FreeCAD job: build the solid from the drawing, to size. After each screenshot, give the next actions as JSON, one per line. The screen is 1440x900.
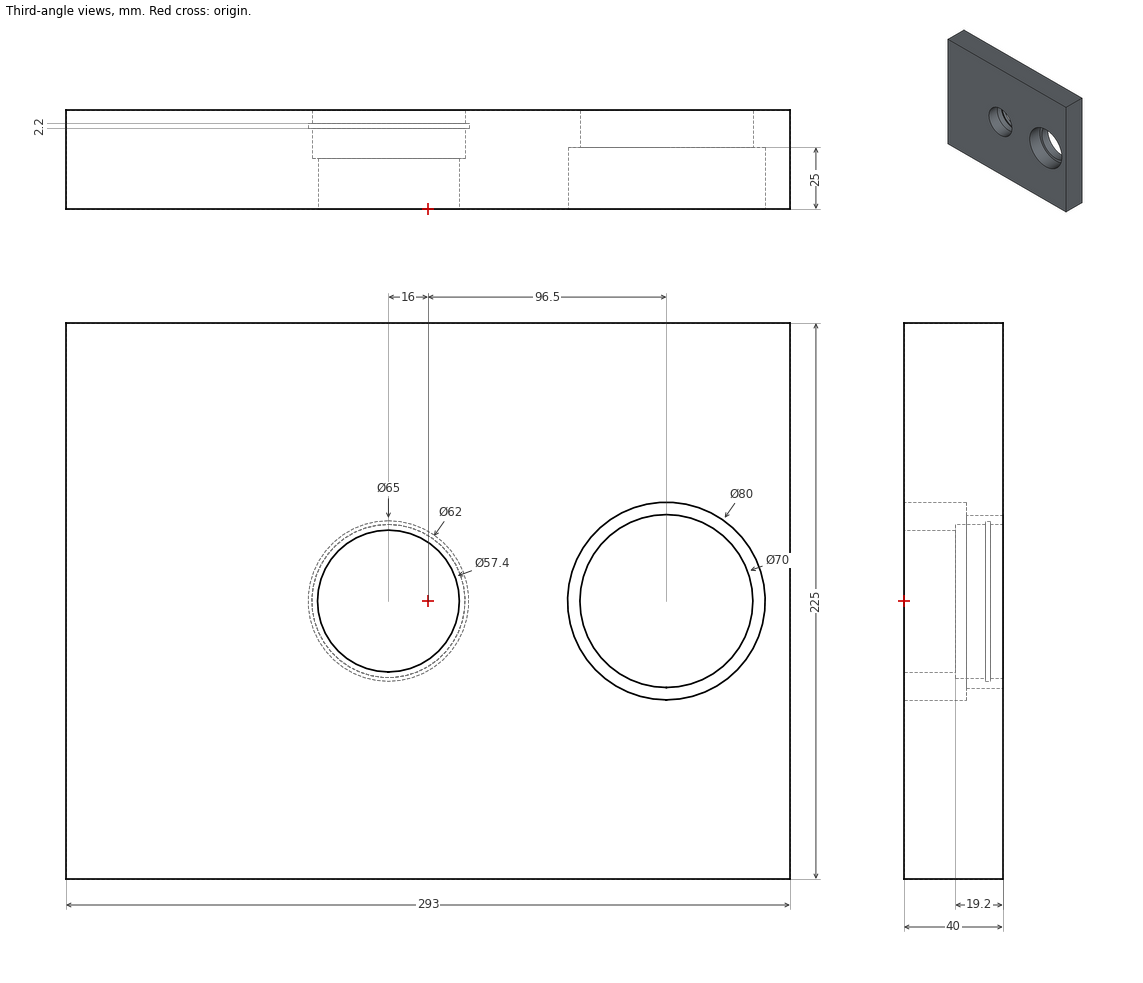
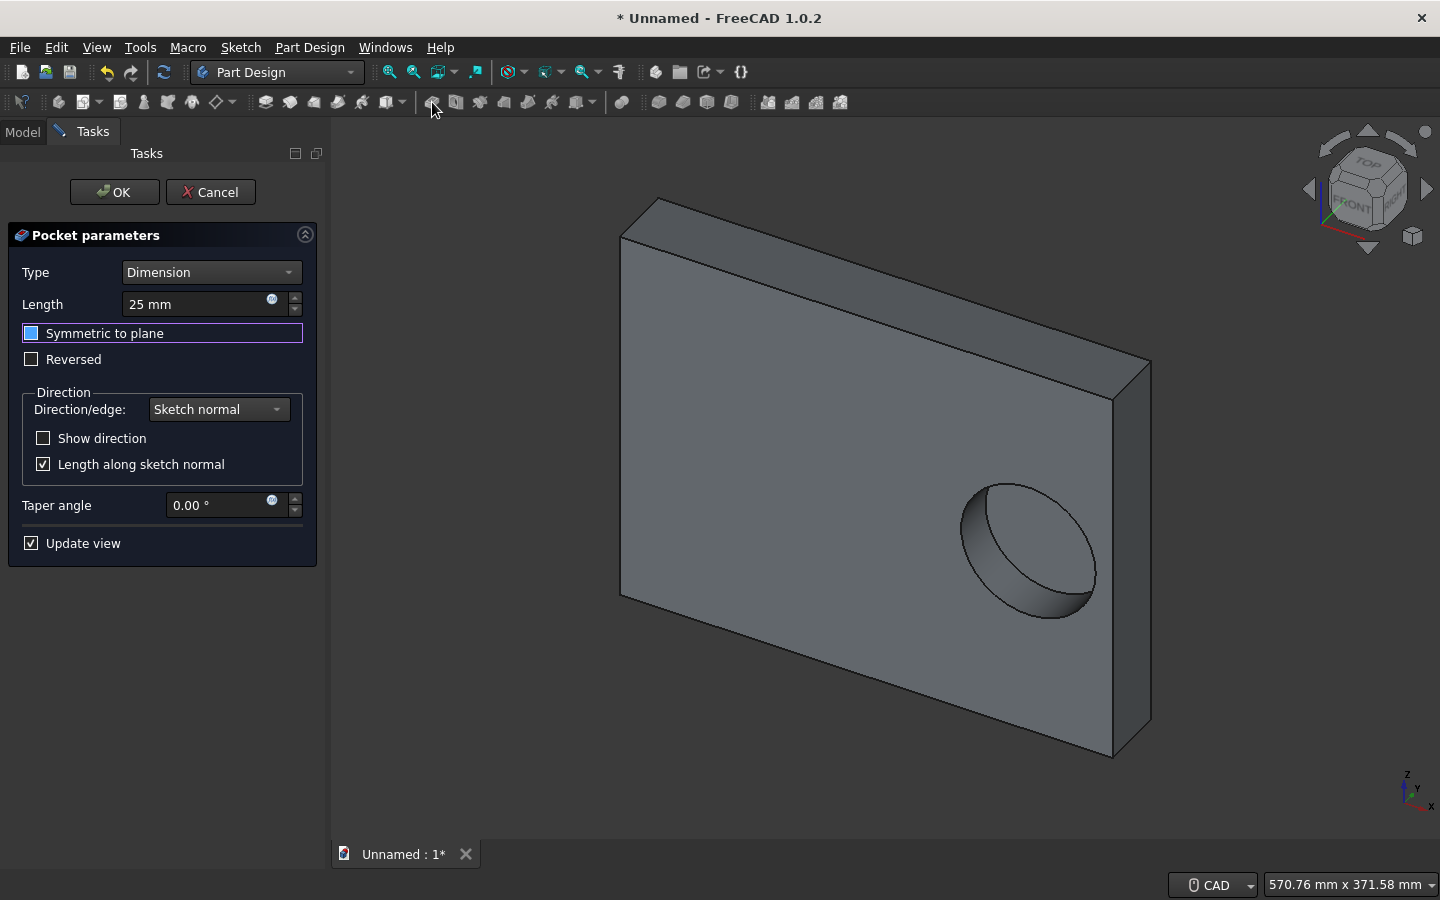
{"action": "left_click", "coordinate": [115, 192]}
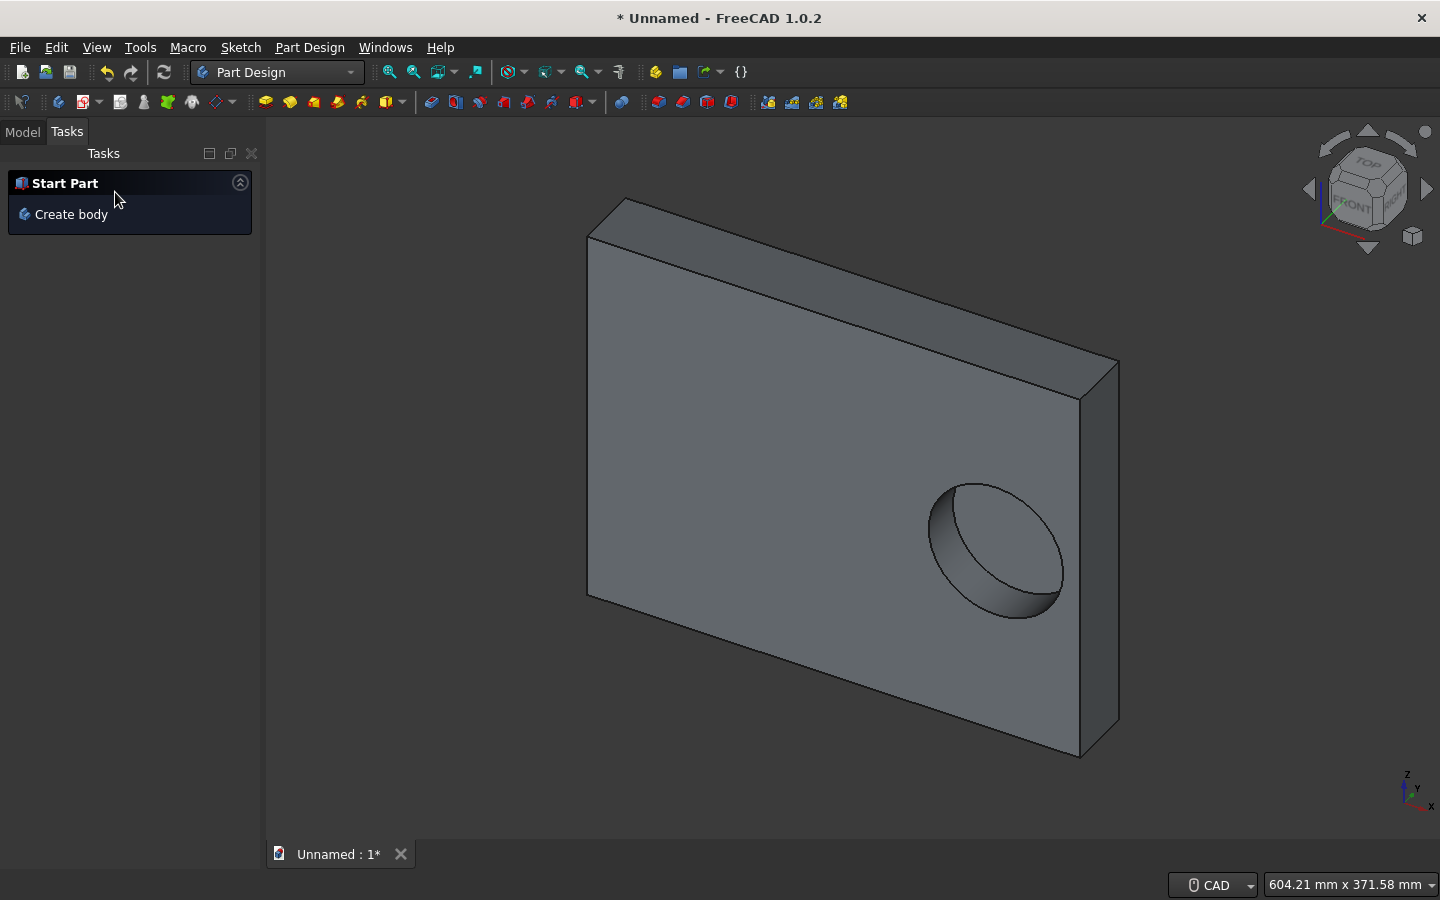
{"action": "left_click", "coordinate": [763, 473]}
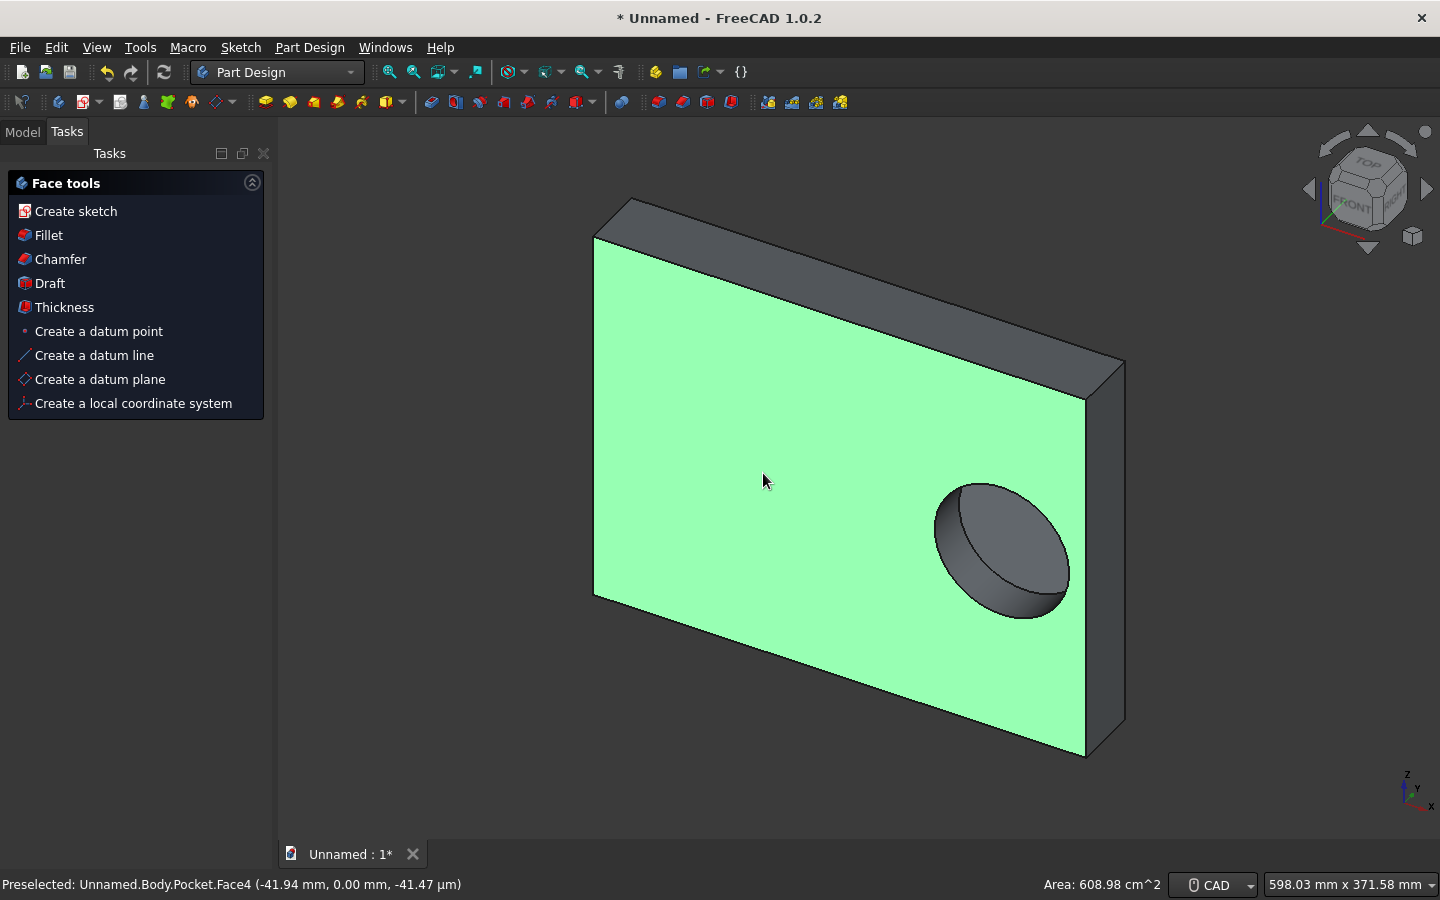
{"action": "left_click", "coordinate": [84, 102]}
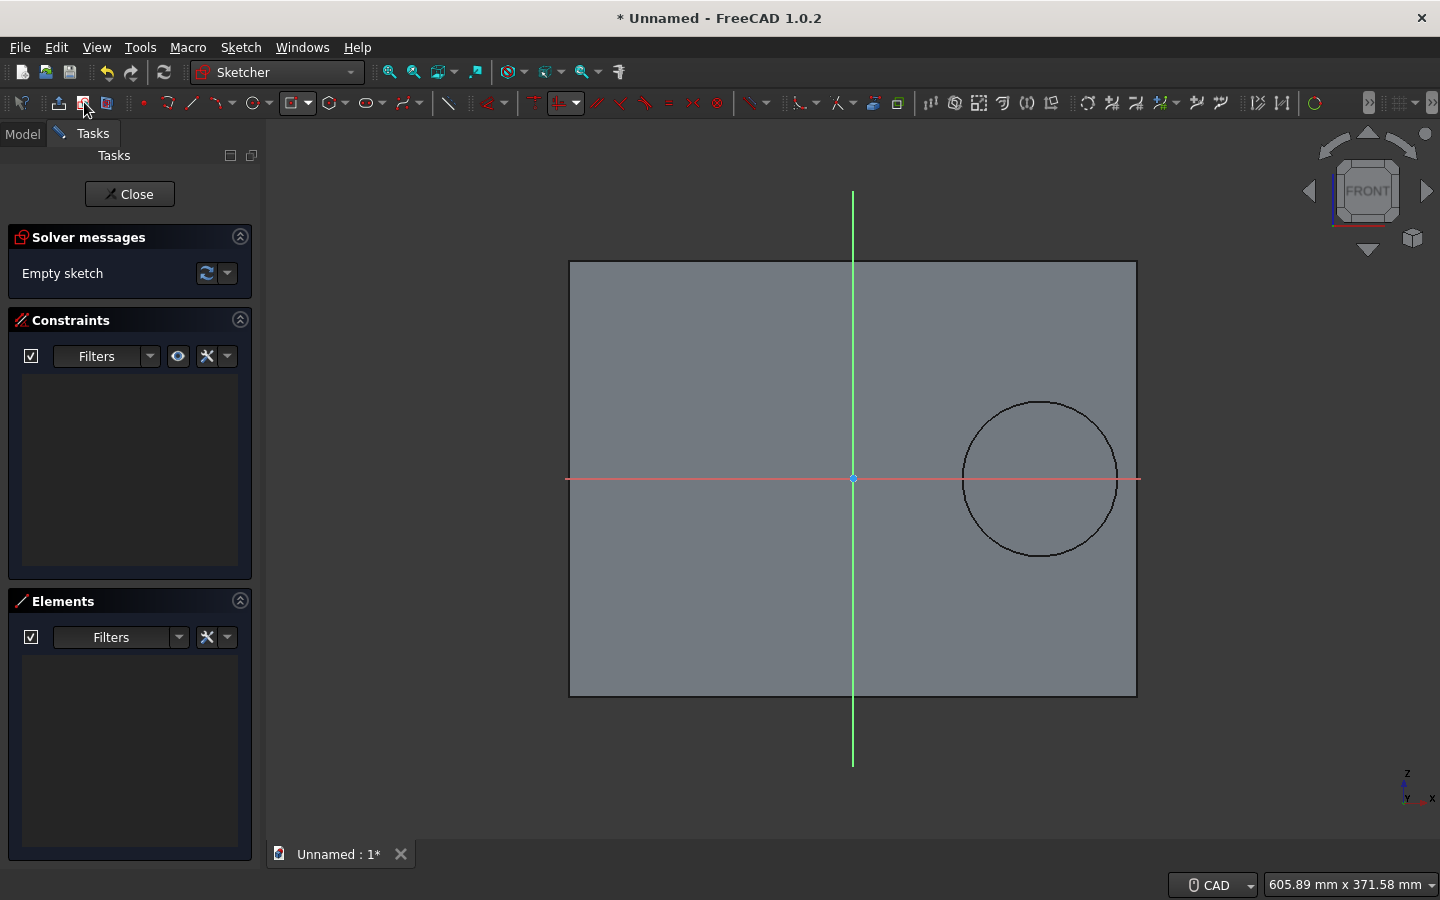
{"action": "scroll", "coordinate": [834, 479], "scroll_direction": "up", "scroll_amount": 7}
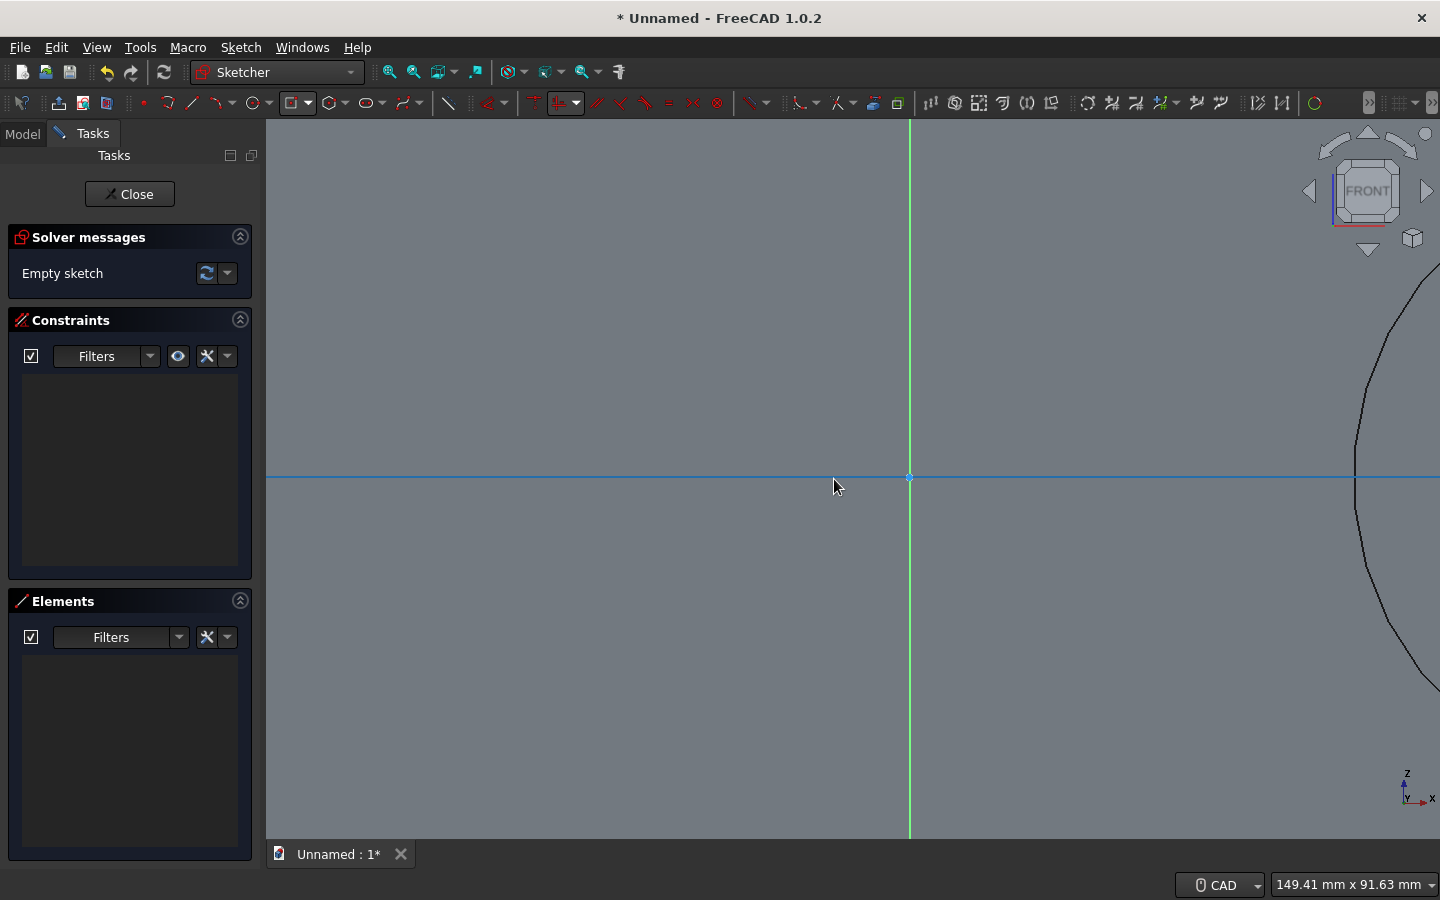
{"action": "left_click", "coordinate": [254, 104]}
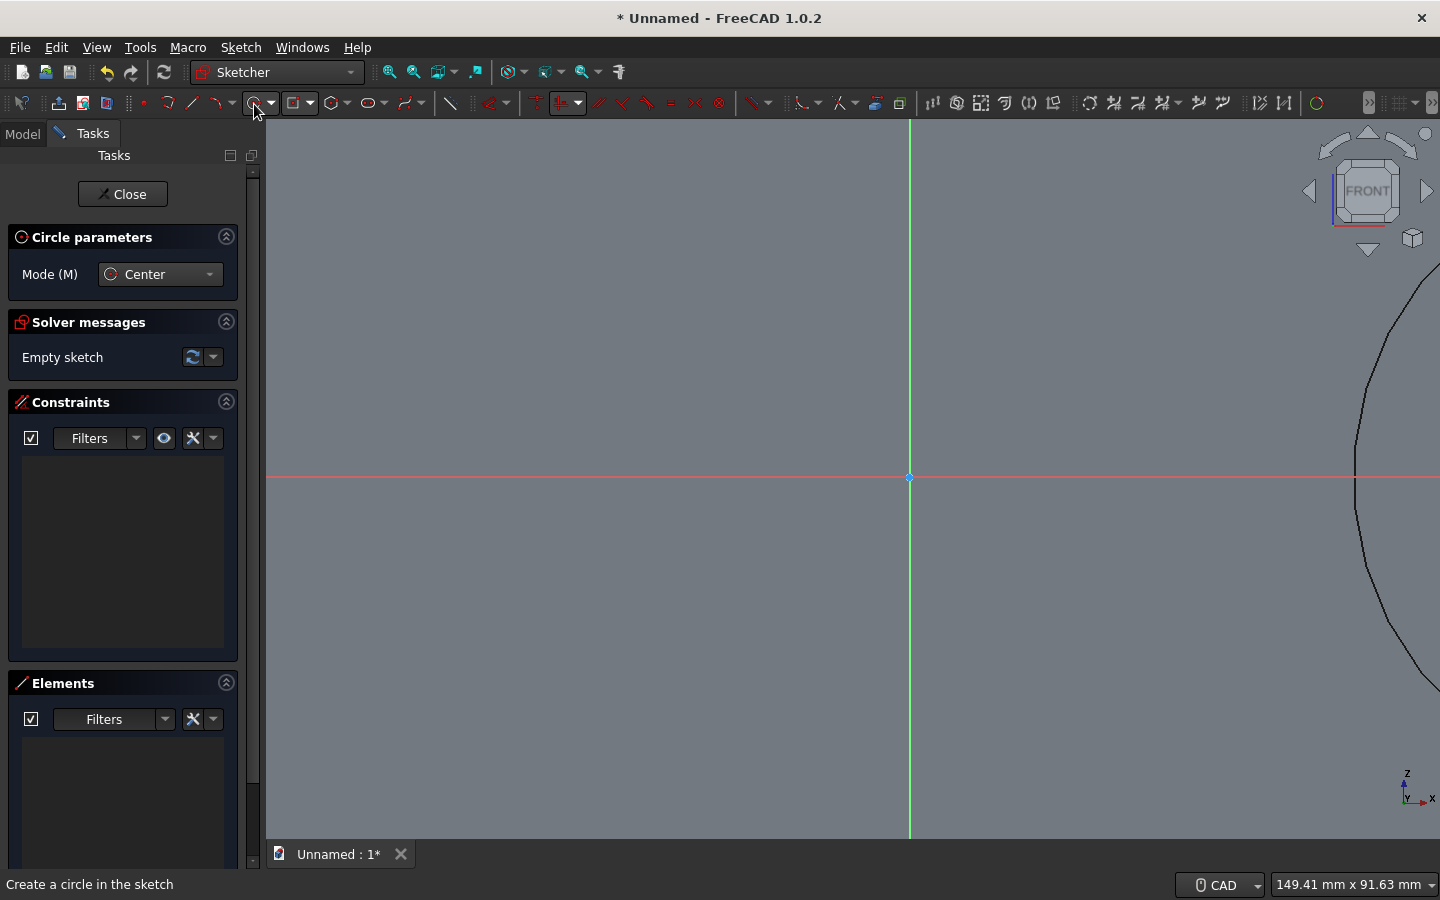
{"action": "left_click", "coordinate": [784, 477]}
{"action": "mouse_move", "coordinate": [943, 318]}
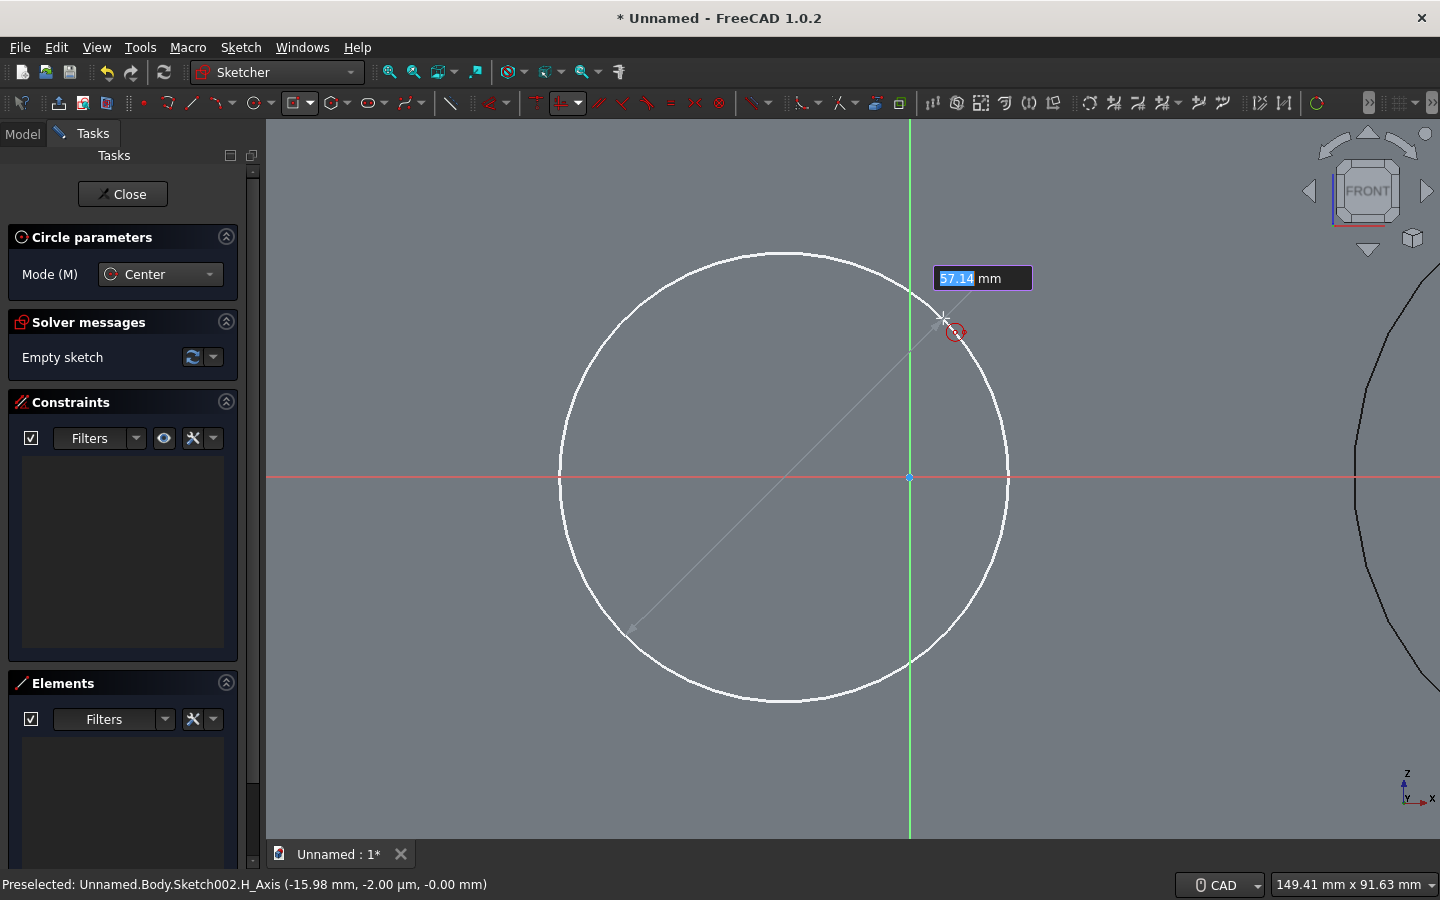
{"action": "type", "text": "57.4"}
{"action": "key", "text": "Return"}
{"action": "key", "text": "Escape"}